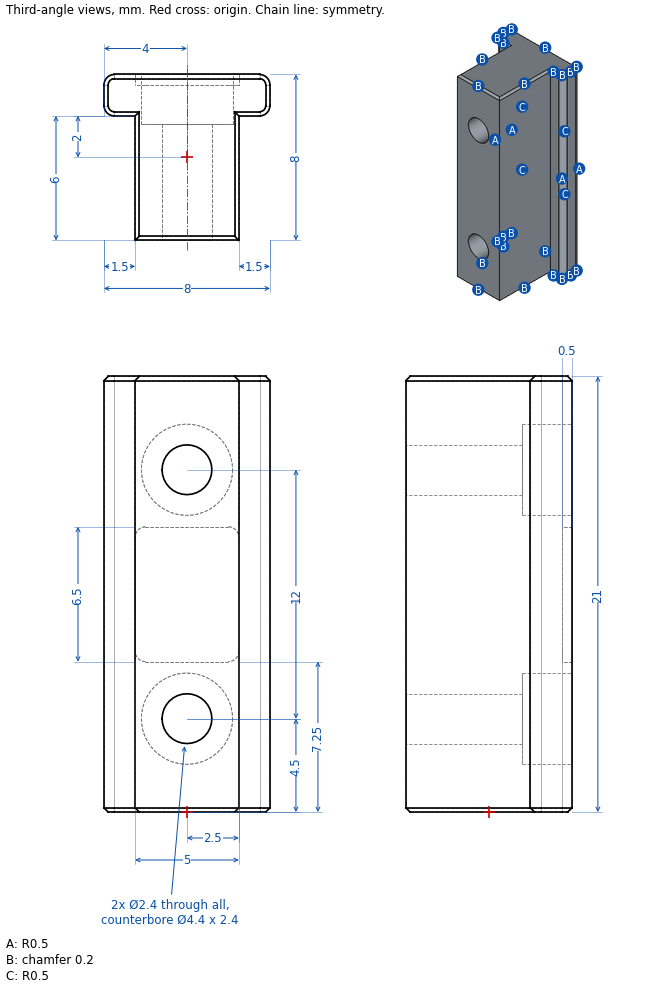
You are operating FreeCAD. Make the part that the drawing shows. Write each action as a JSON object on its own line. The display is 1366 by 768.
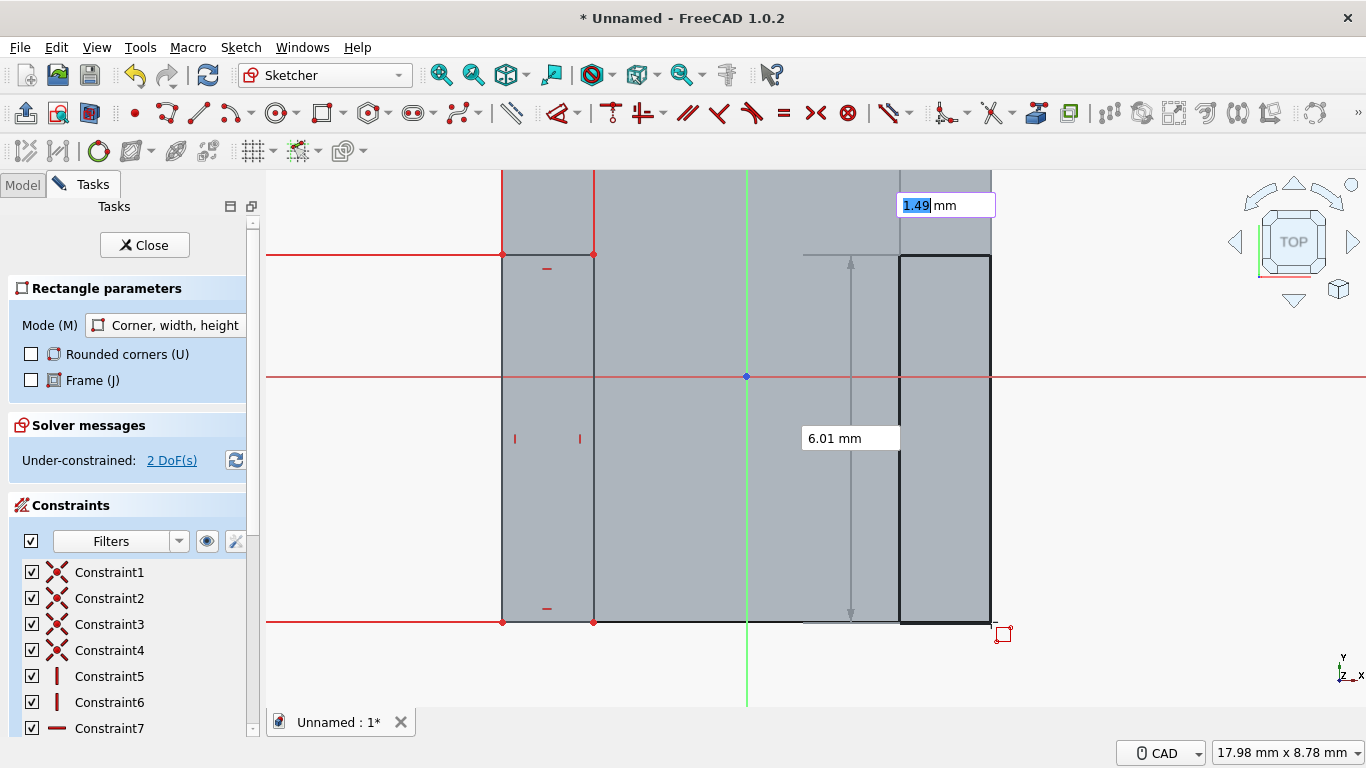
{"action": "type", "text": "1.5"}
{"action": "key", "text": "Tab"}
{"action": "type", "text": "6"}
{"action": "key", "text": "Return"}
{"action": "key", "text": "Escape"}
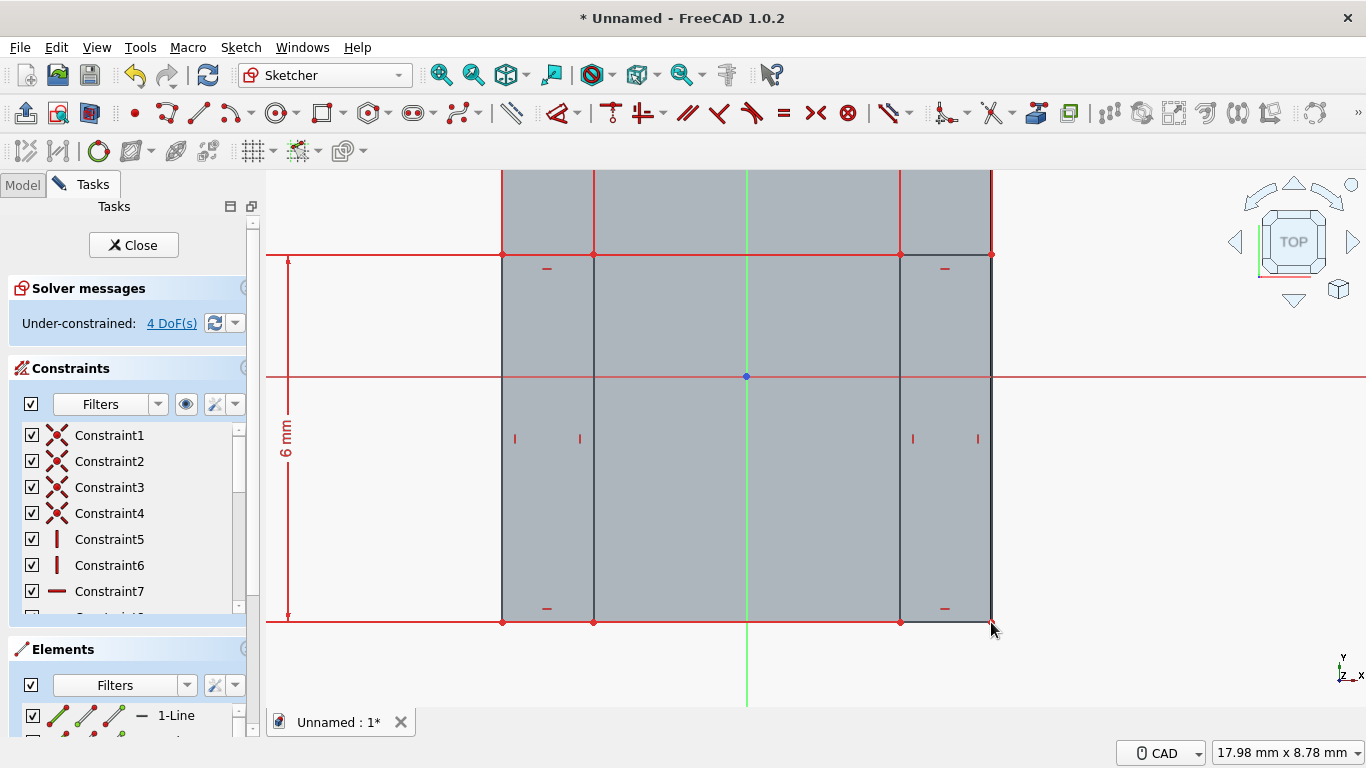
{"action": "left_click", "coordinate": [594, 255]}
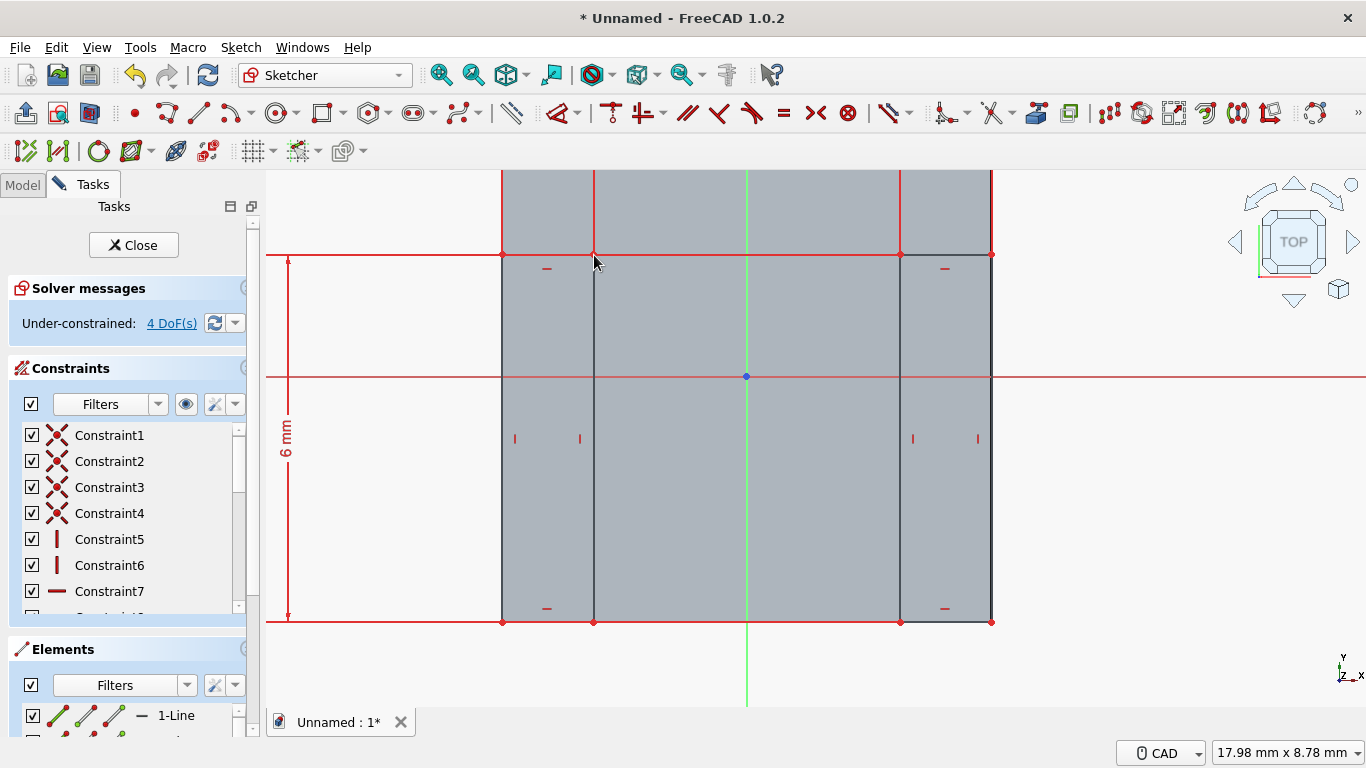
{"action": "left_click", "coordinate": [900, 255]}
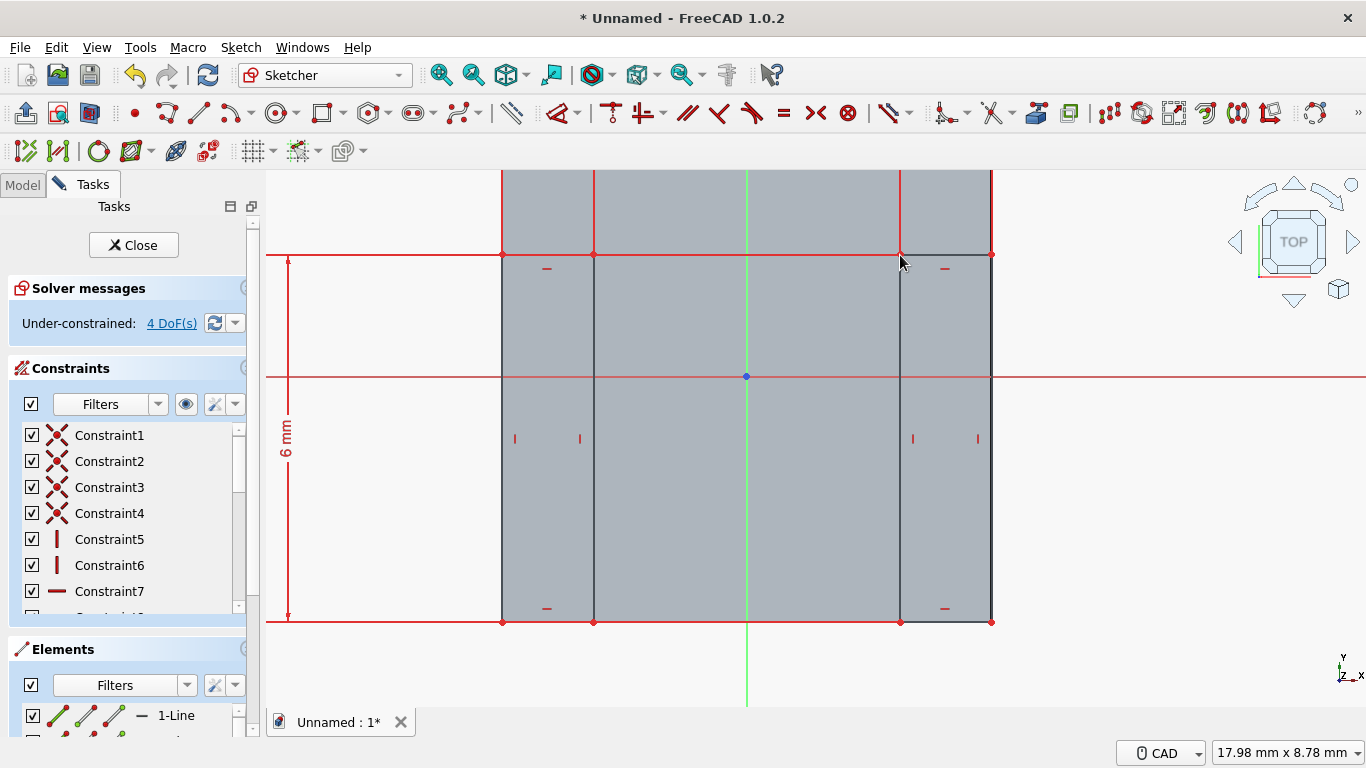
{"action": "left_click", "coordinate": [747, 645]}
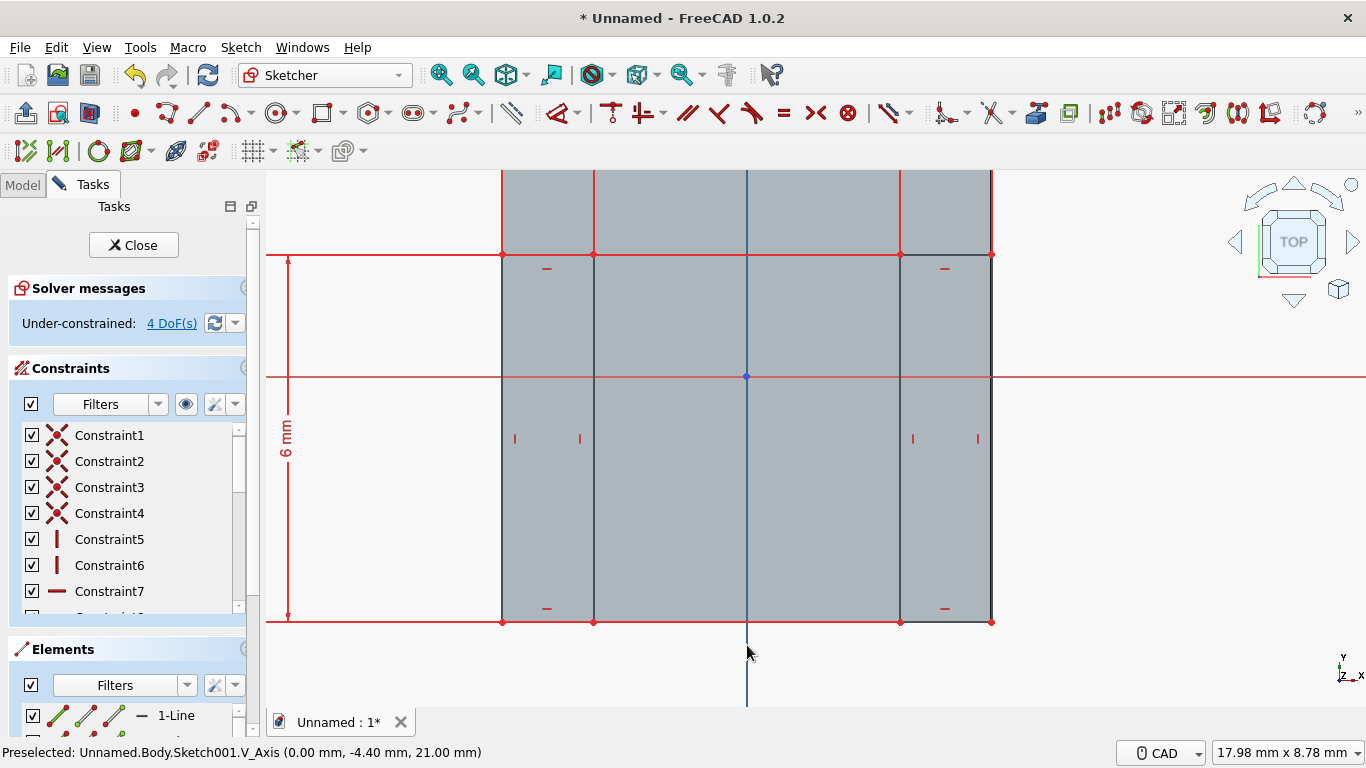
{"action": "left_click", "coordinate": [816, 114]}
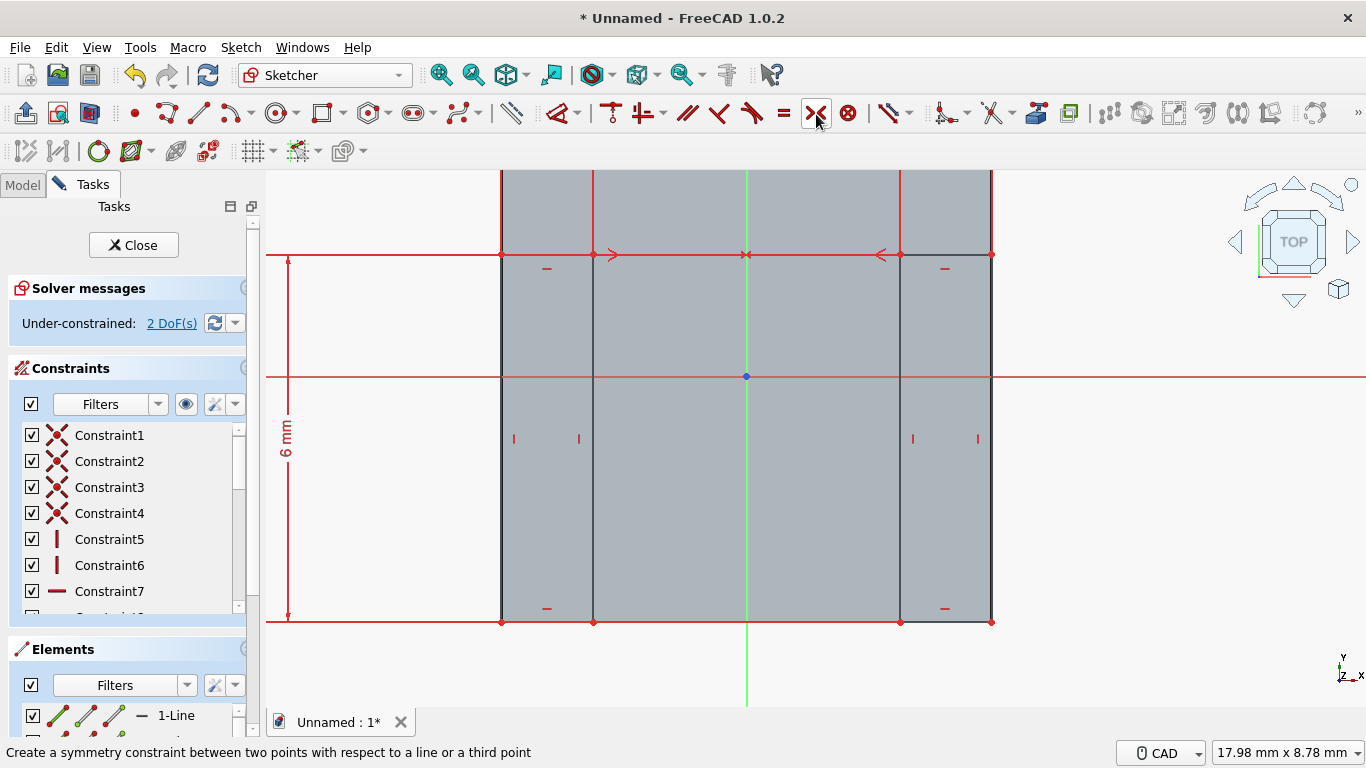
{"action": "left_click", "coordinate": [558, 114]}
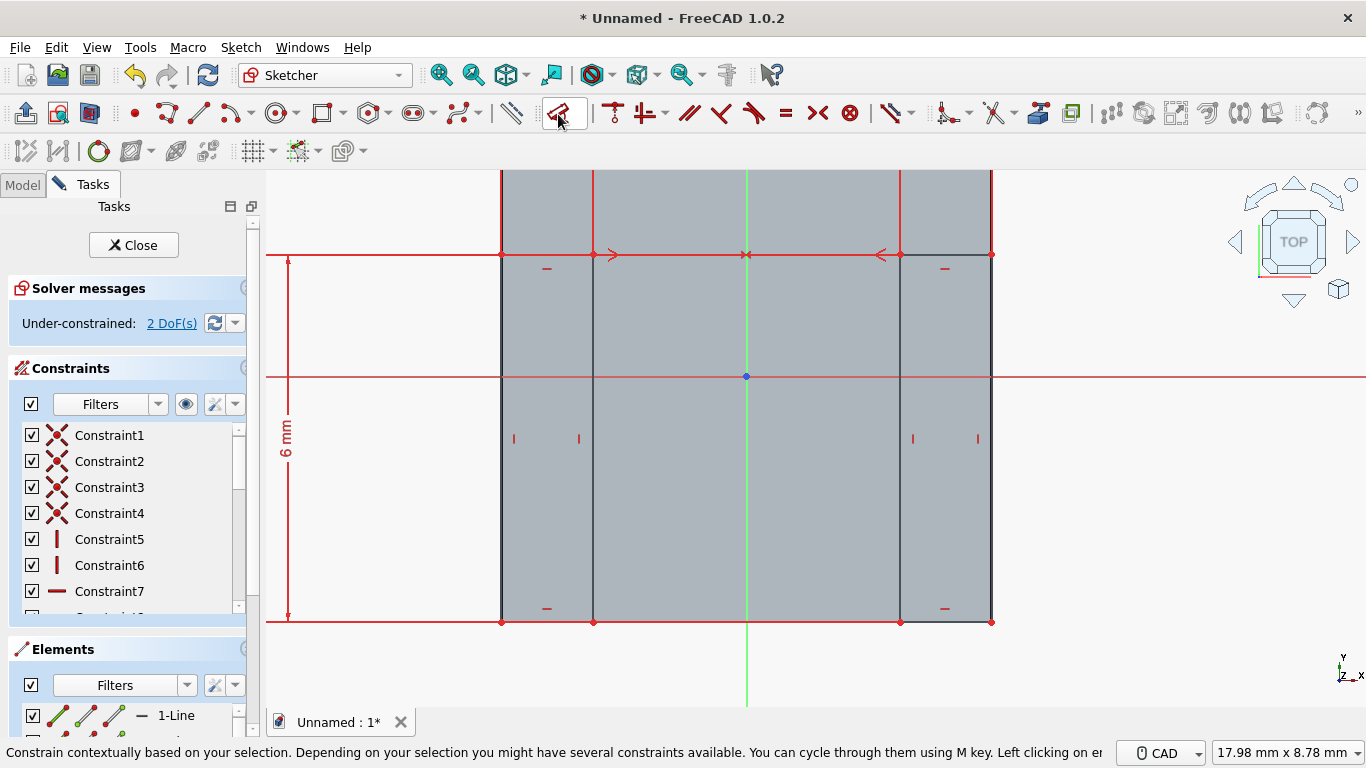
{"action": "left_click", "coordinate": [501, 255]}
{"action": "left_click", "coordinate": [624, 221]}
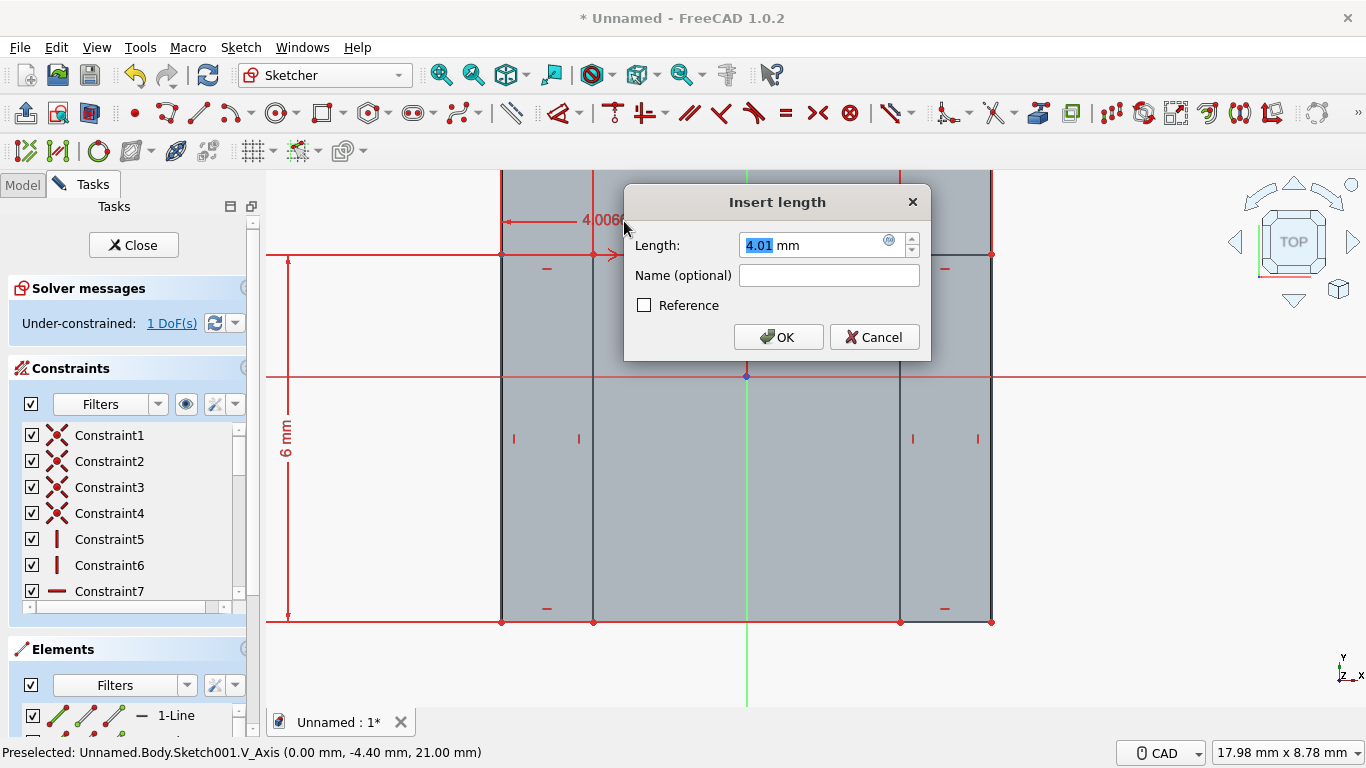
{"action": "type", "text": "4"}
{"action": "key", "text": "Return"}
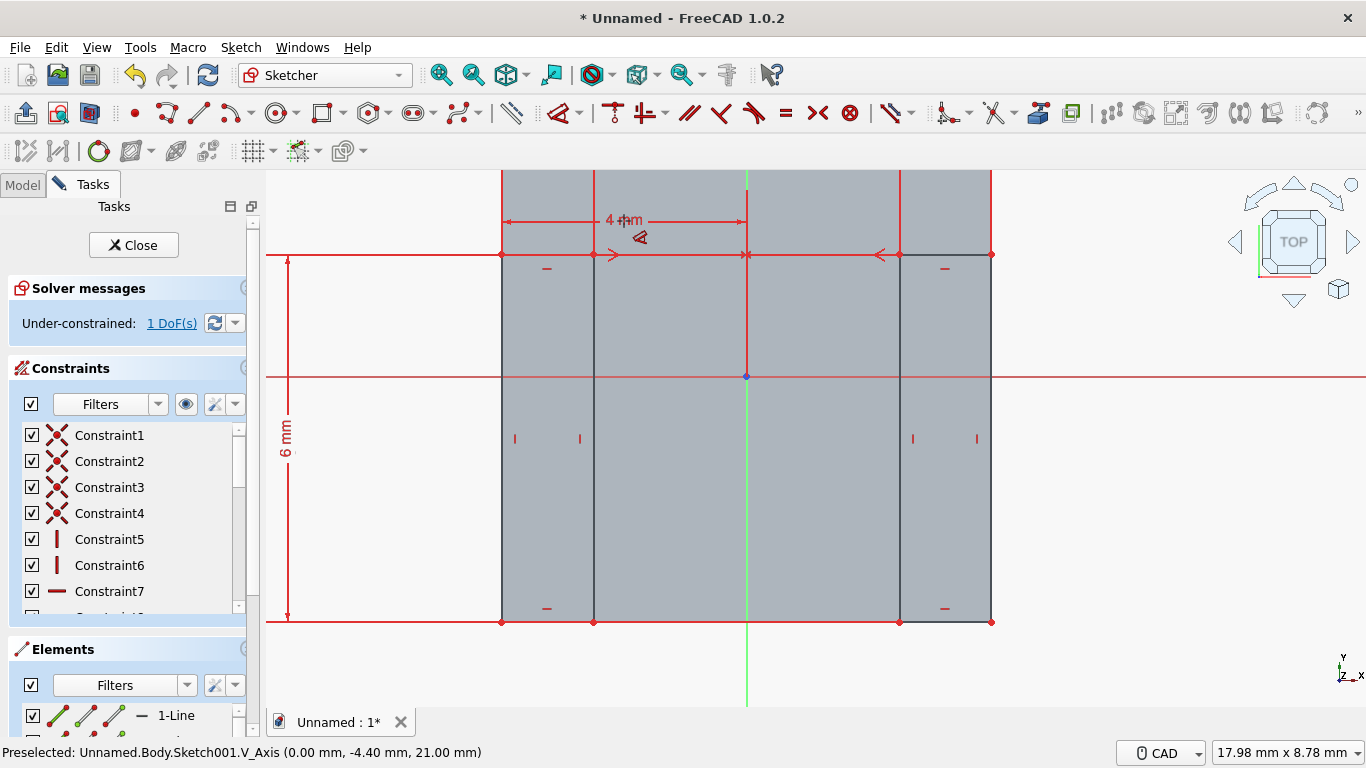
{"action": "left_click", "coordinate": [502, 255]}
{"action": "left_click", "coordinate": [468, 316]}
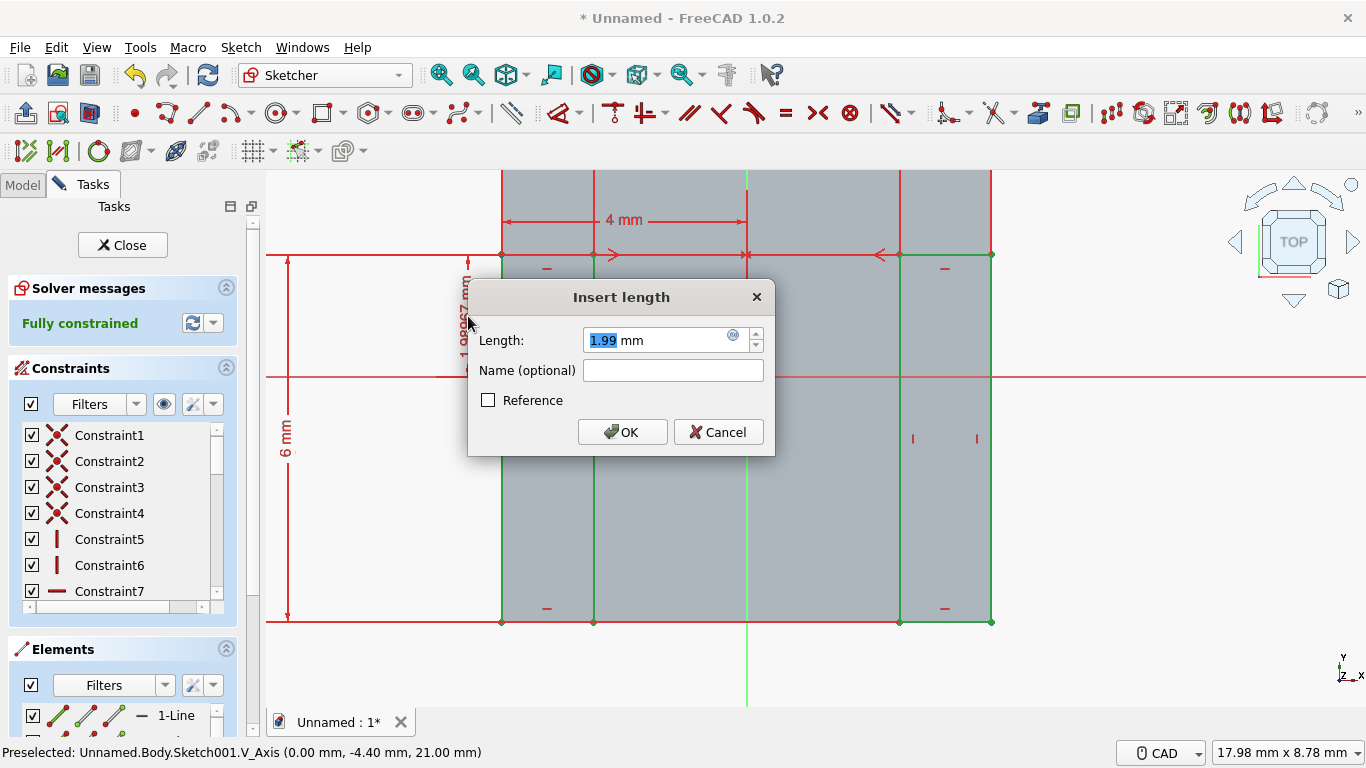
{"action": "type", "text": "2"}
{"action": "key", "text": "Return"}
{"action": "key", "text": "Escape"}